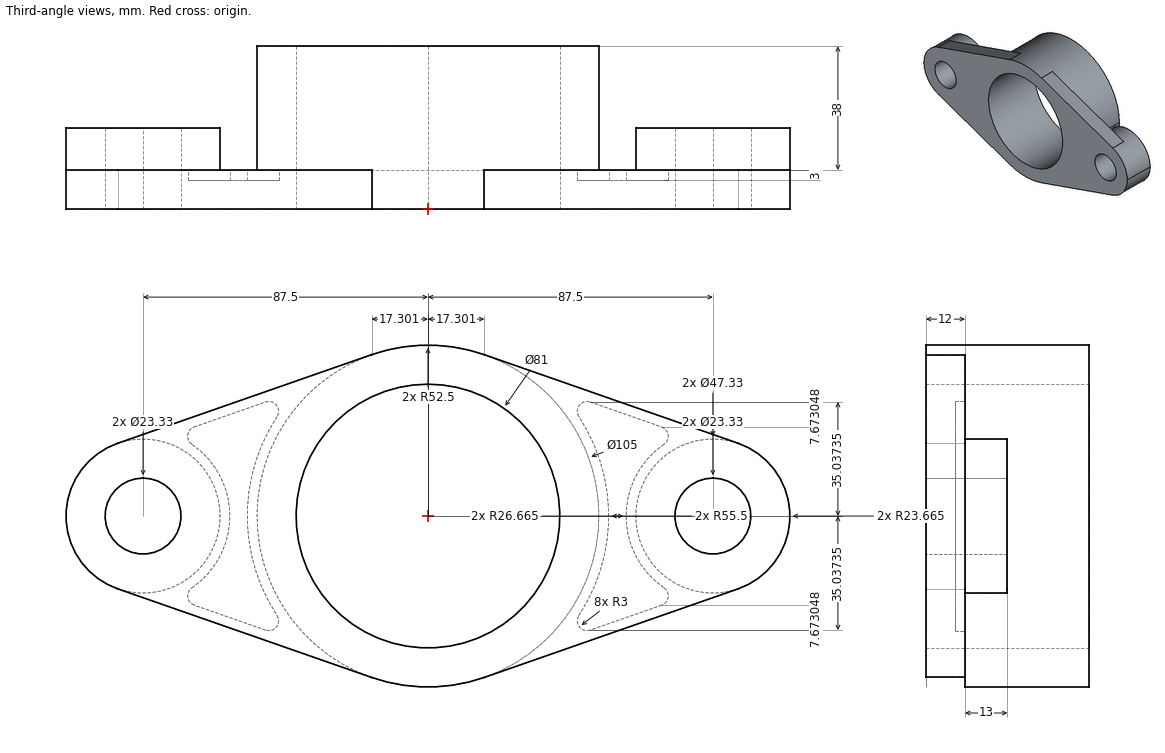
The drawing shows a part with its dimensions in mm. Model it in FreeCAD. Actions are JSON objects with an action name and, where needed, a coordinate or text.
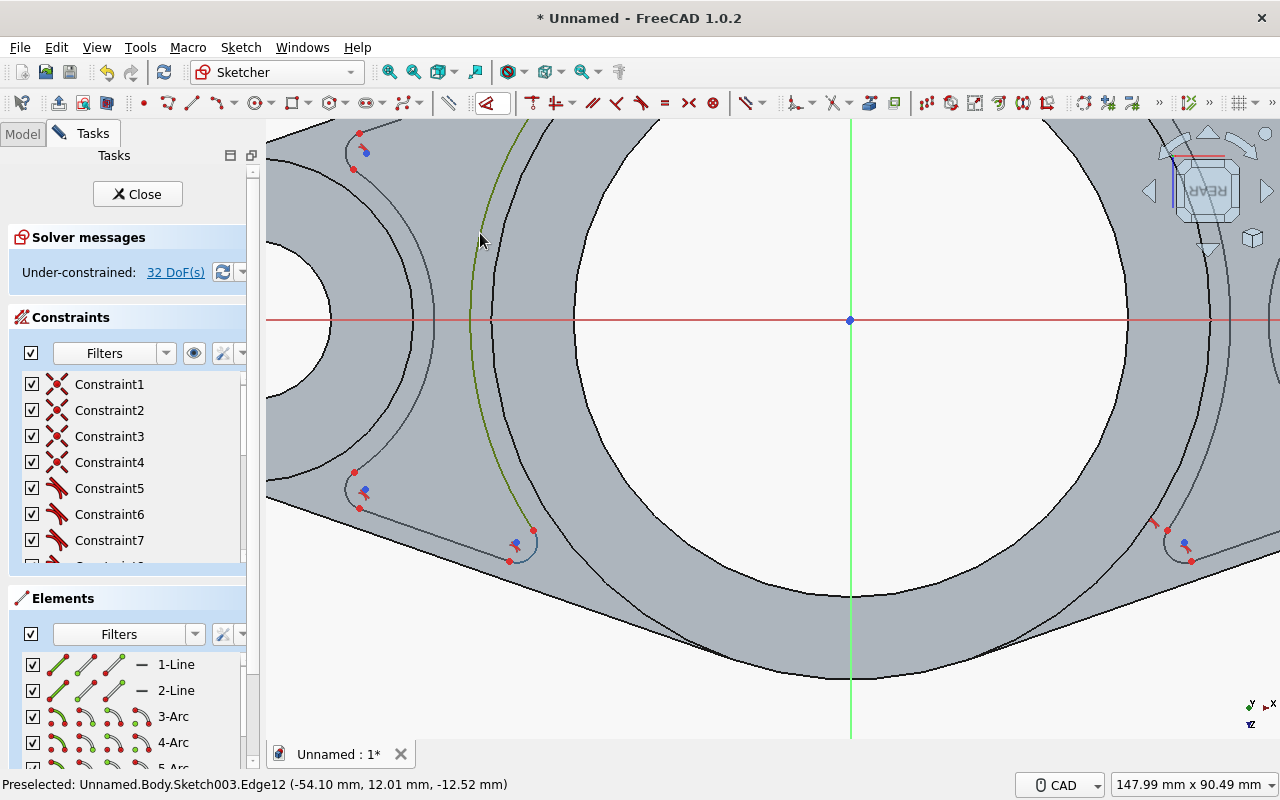
{"action": "left_click", "coordinate": [642, 104]}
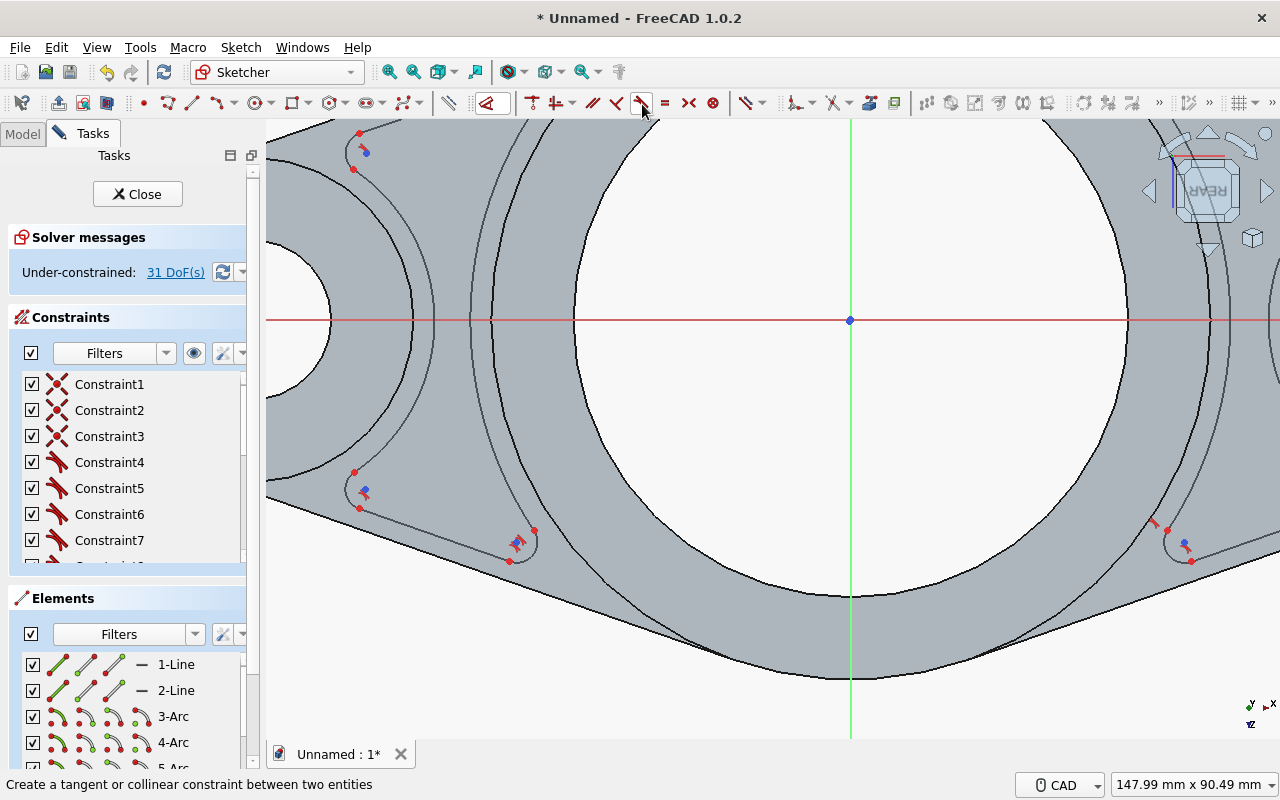
{"action": "left_click", "coordinate": [481, 233]}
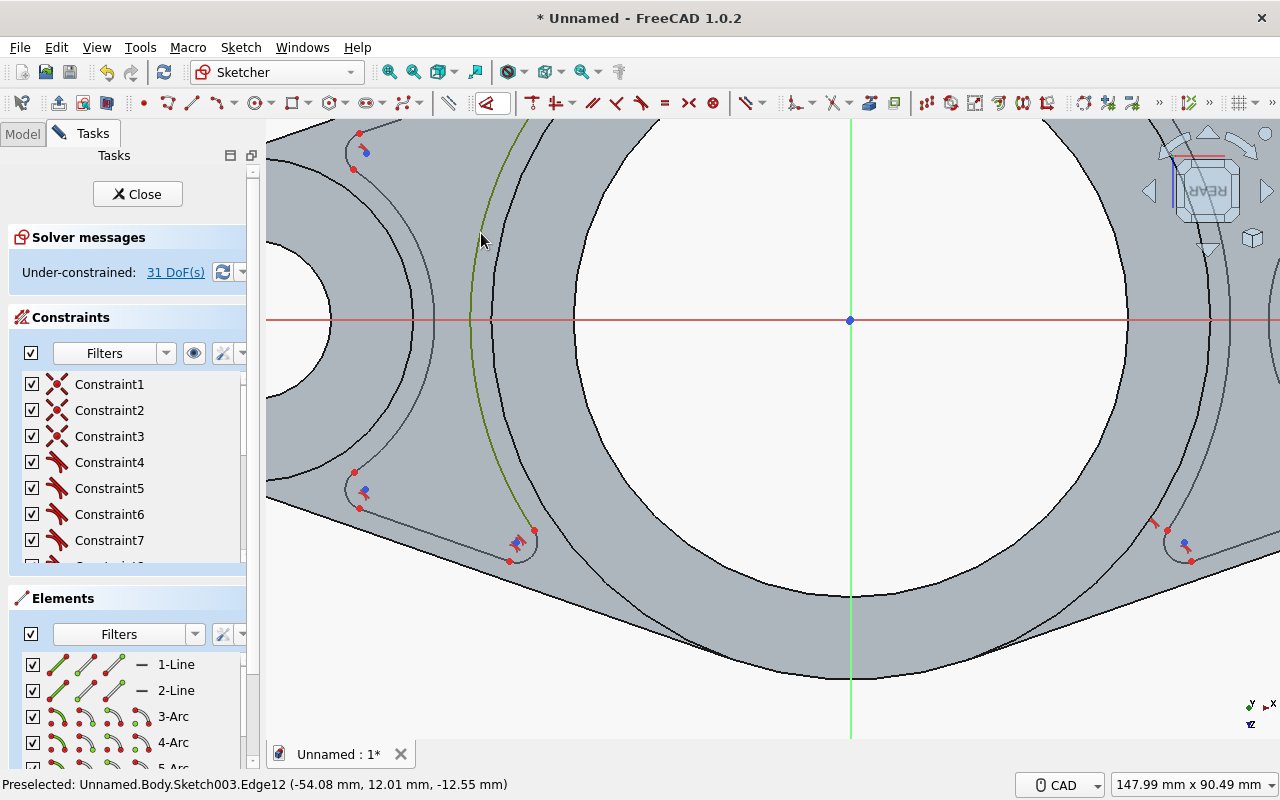
{"action": "scroll", "coordinate": [526, 562], "scroll_direction": "down", "scroll_amount": 3}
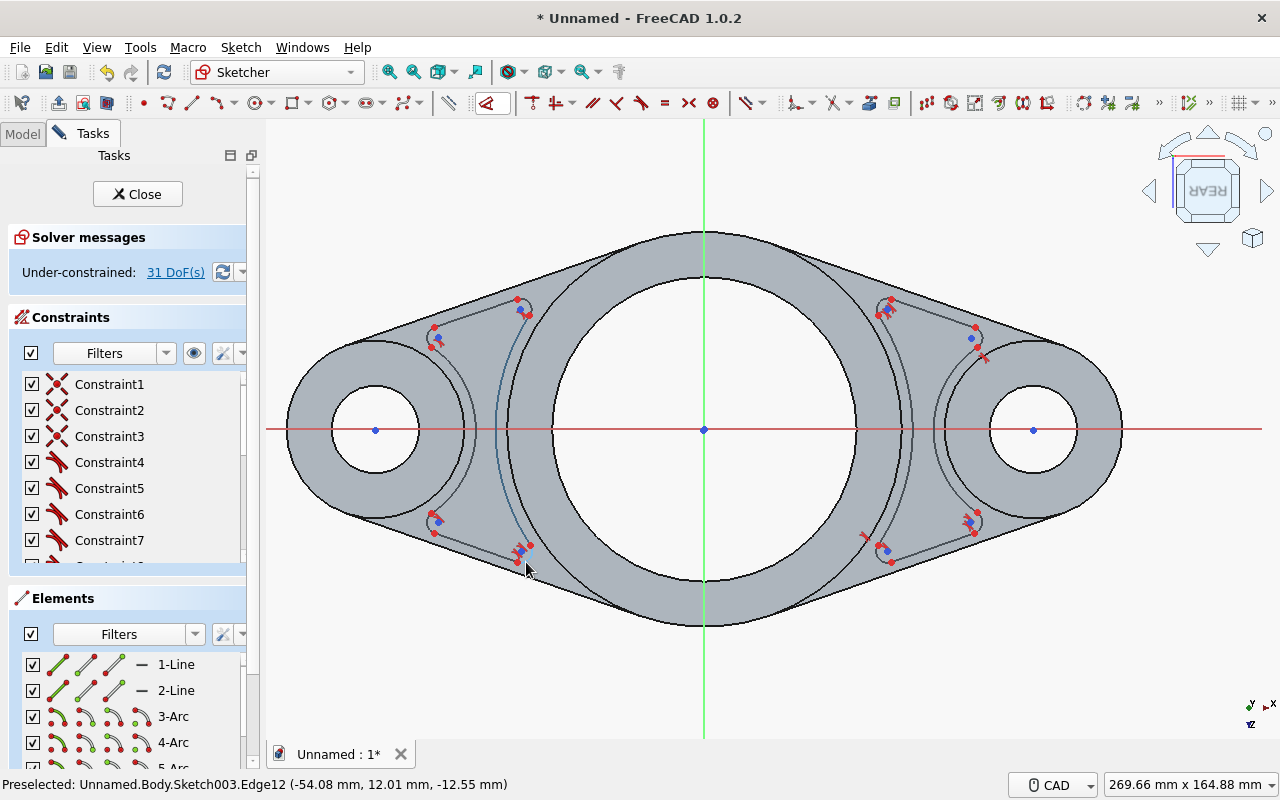
{"action": "scroll", "coordinate": [531, 307], "scroll_direction": "up", "scroll_amount": 3}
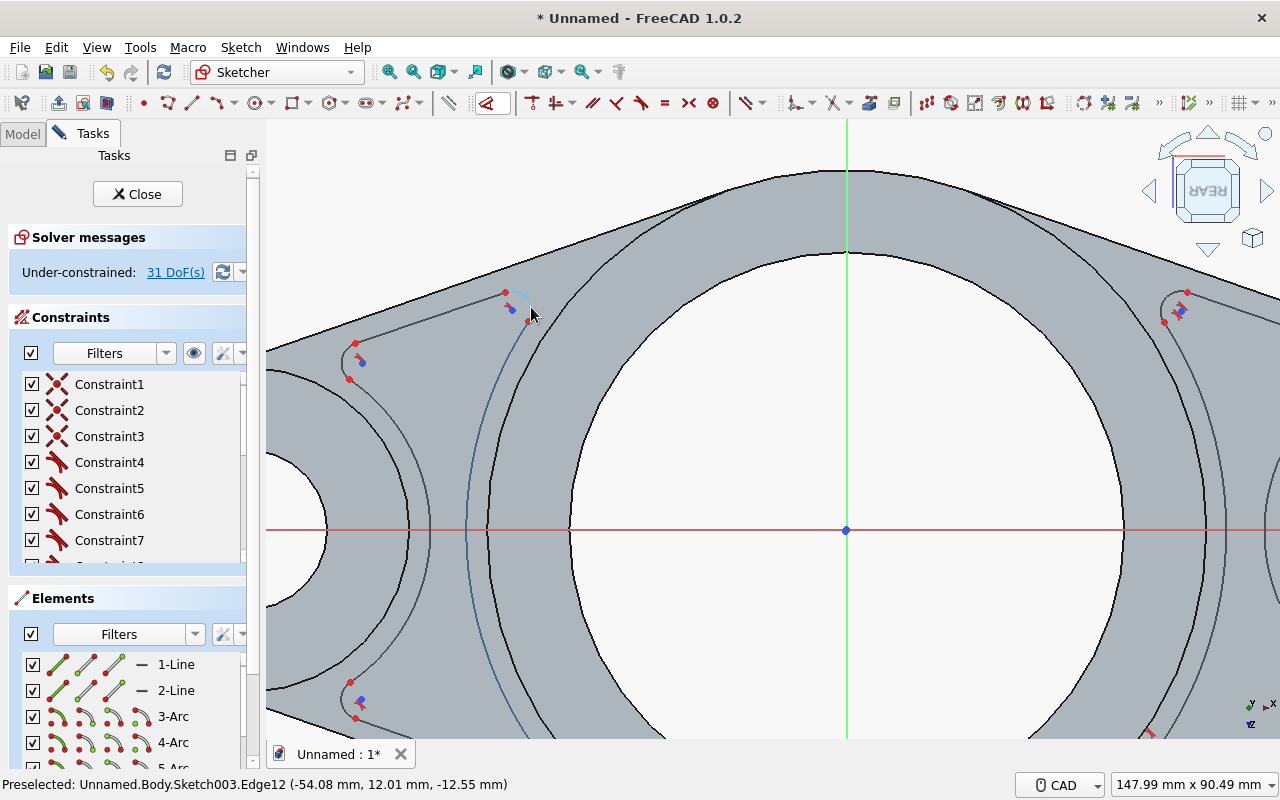
{"action": "left_click", "coordinate": [532, 308]}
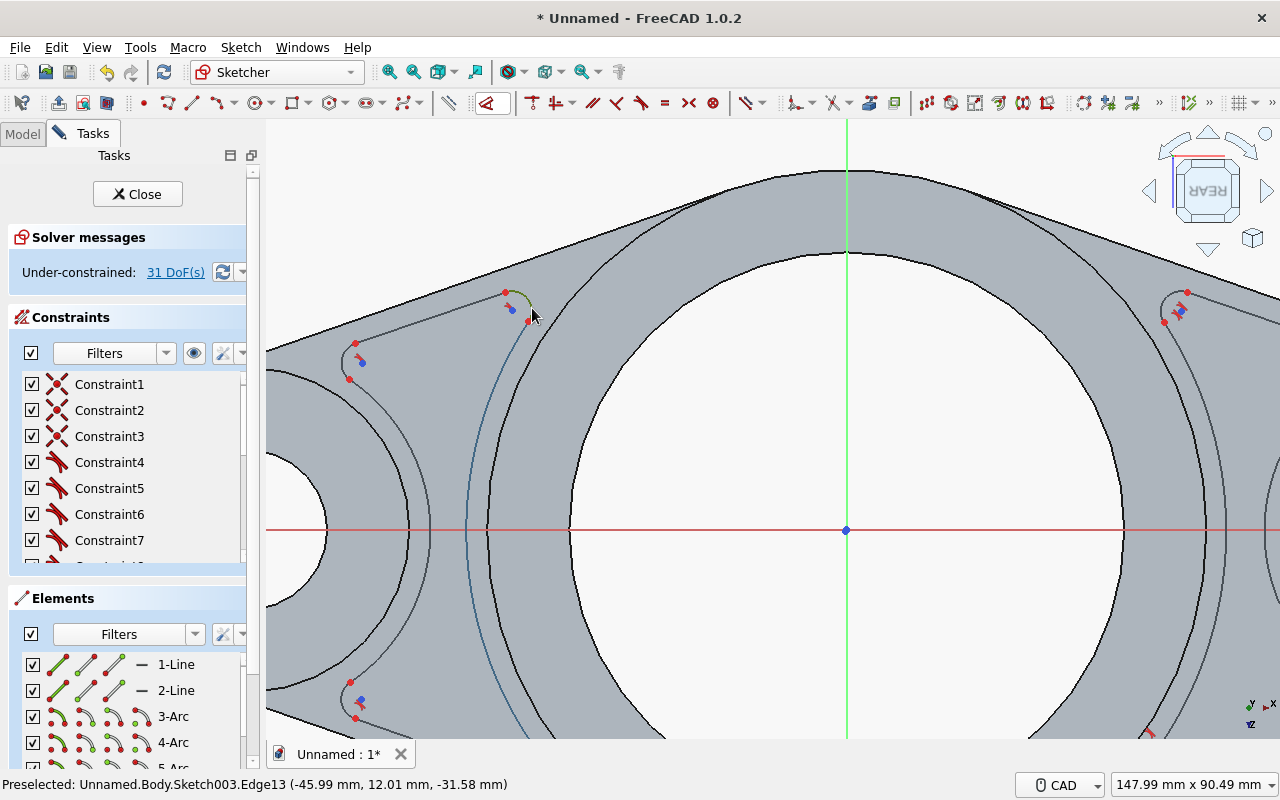
{"action": "left_click", "coordinate": [642, 104]}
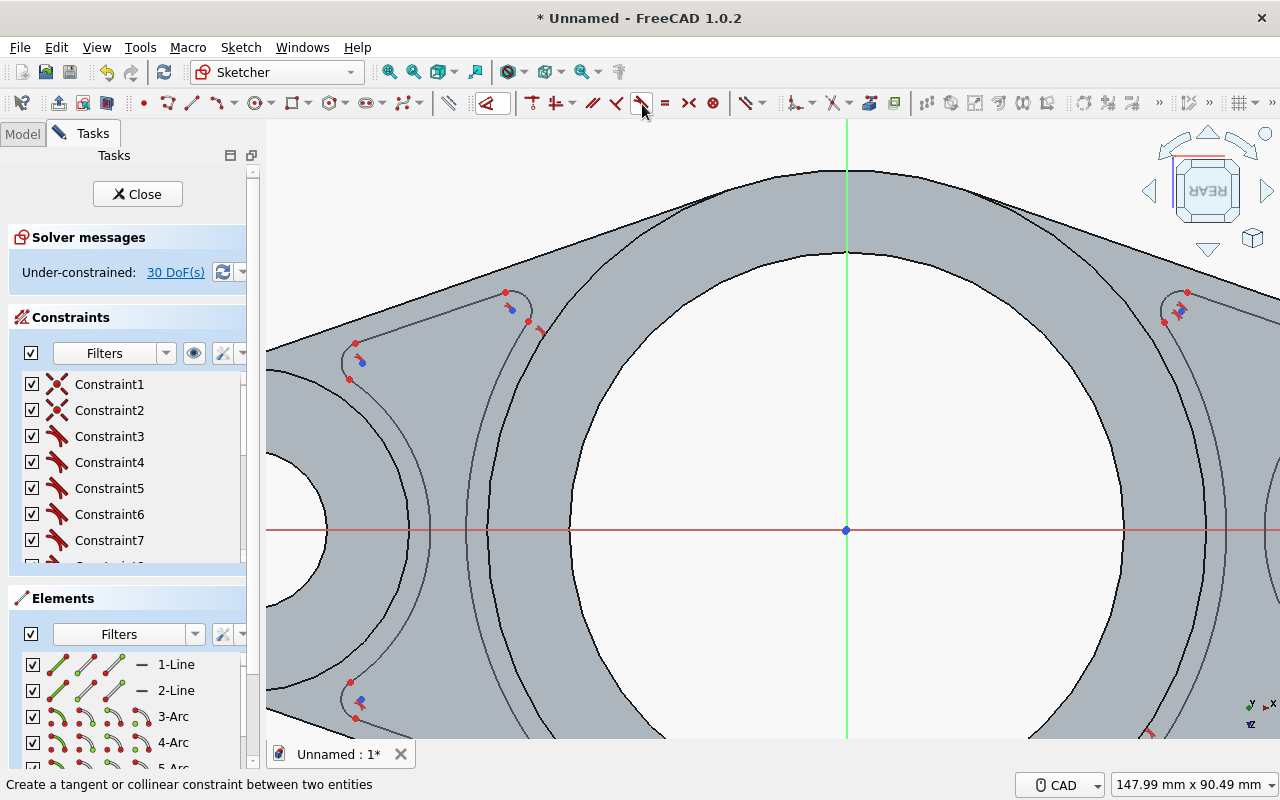
{"action": "left_click", "coordinate": [345, 351]}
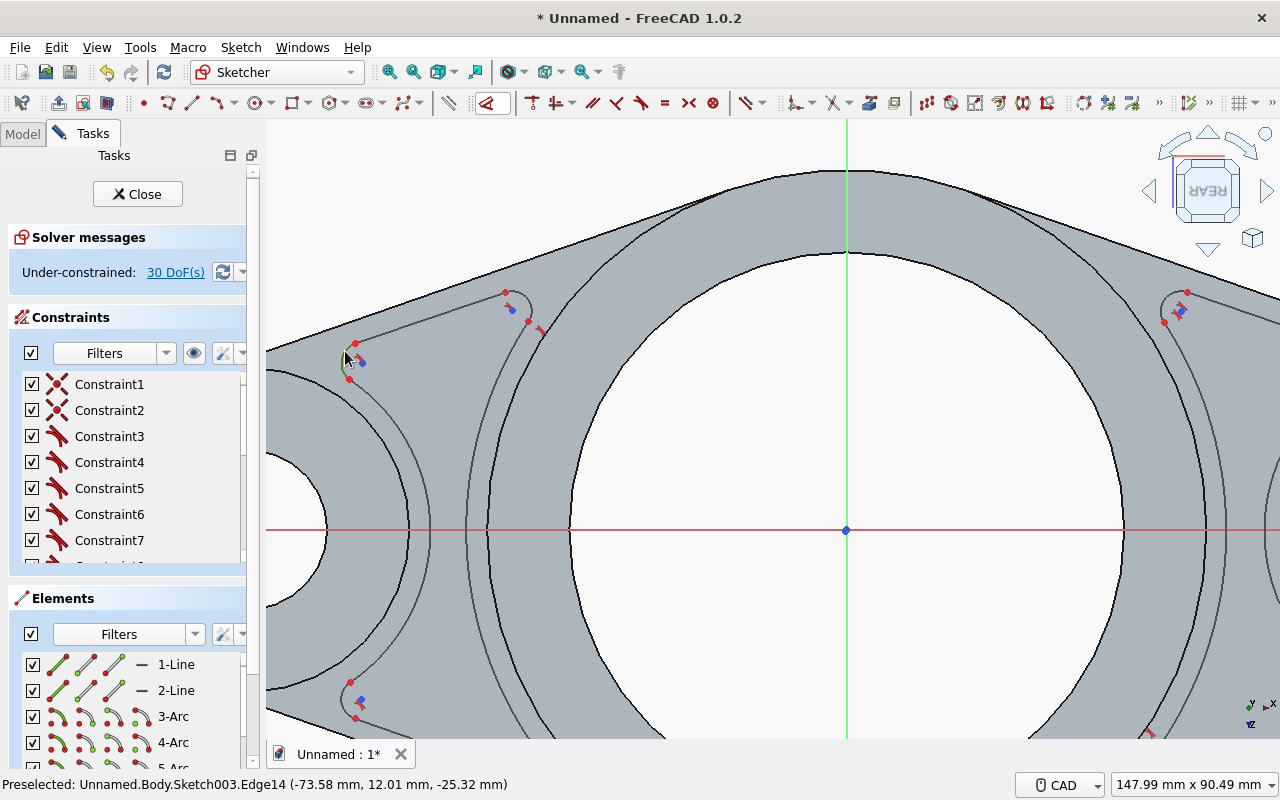
{"action": "left_click", "coordinate": [417, 600]}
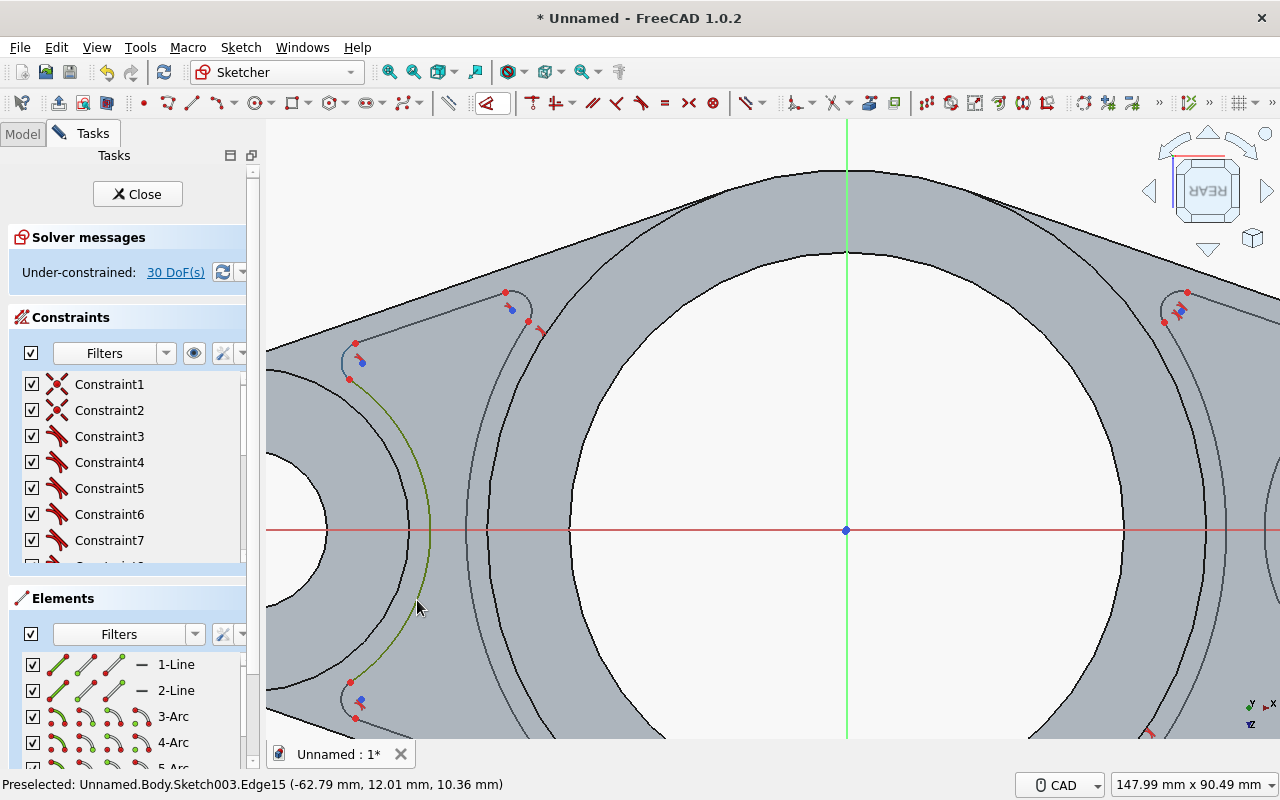
{"action": "left_click", "coordinate": [642, 104]}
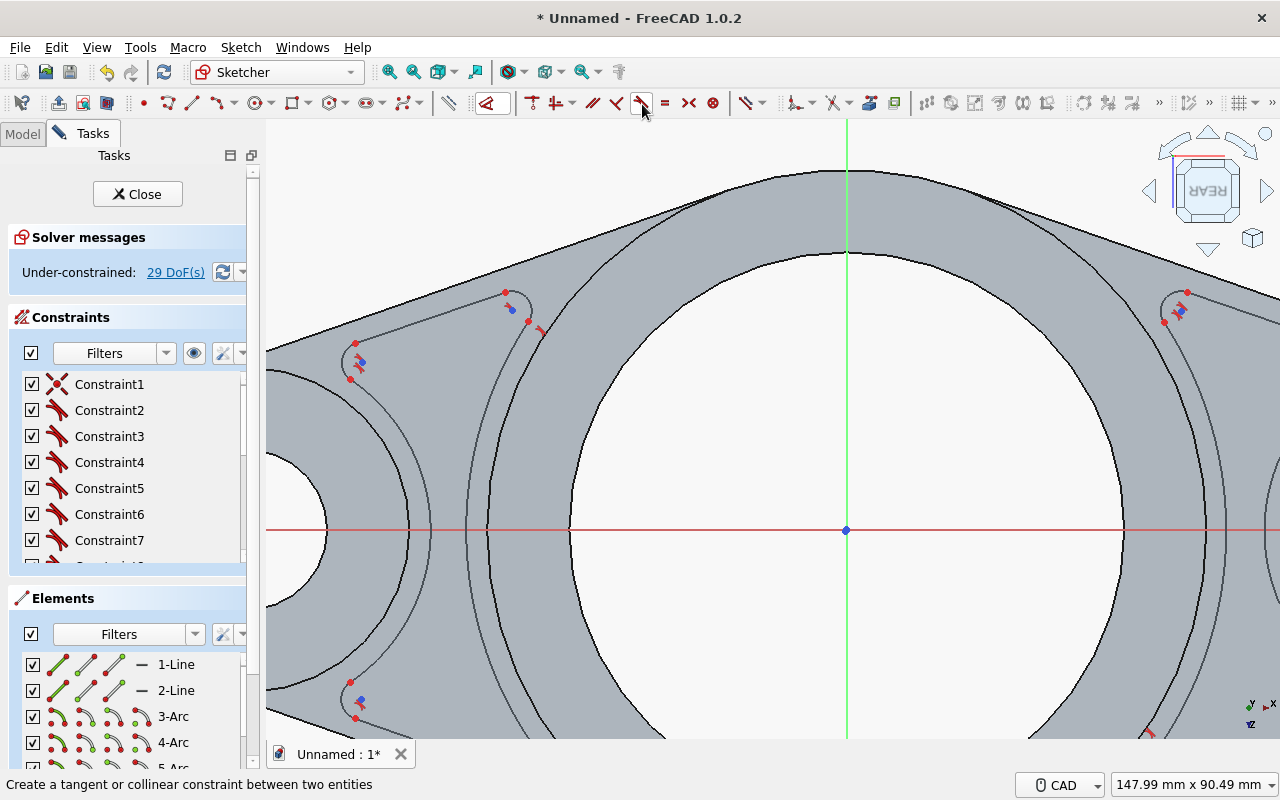
{"action": "left_click", "coordinate": [417, 601]}